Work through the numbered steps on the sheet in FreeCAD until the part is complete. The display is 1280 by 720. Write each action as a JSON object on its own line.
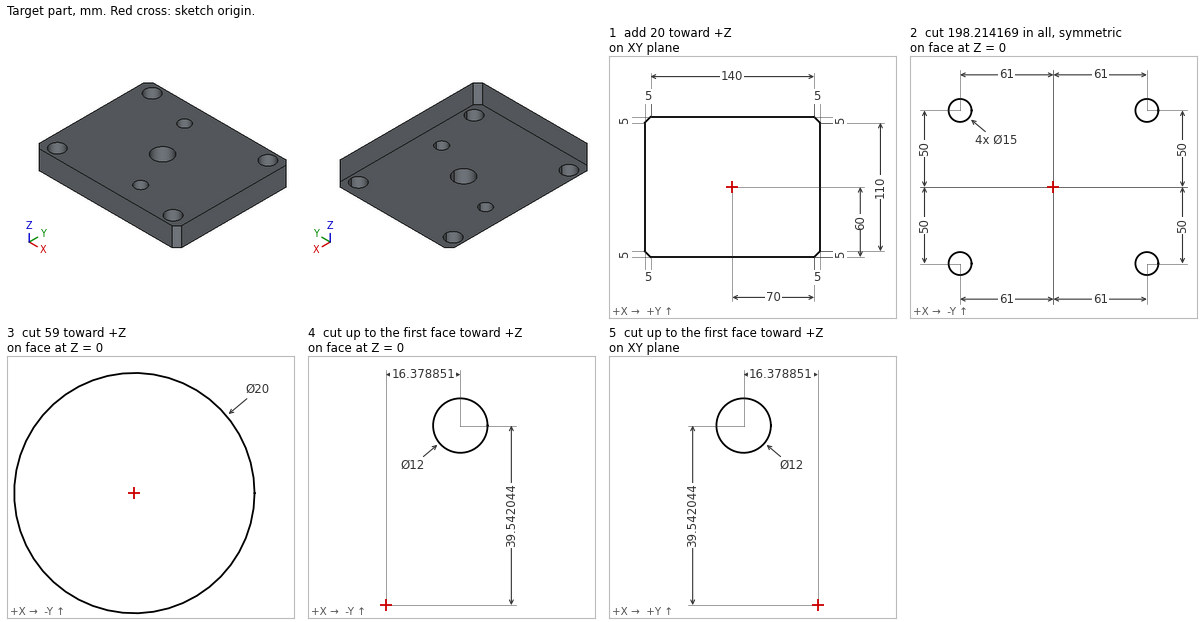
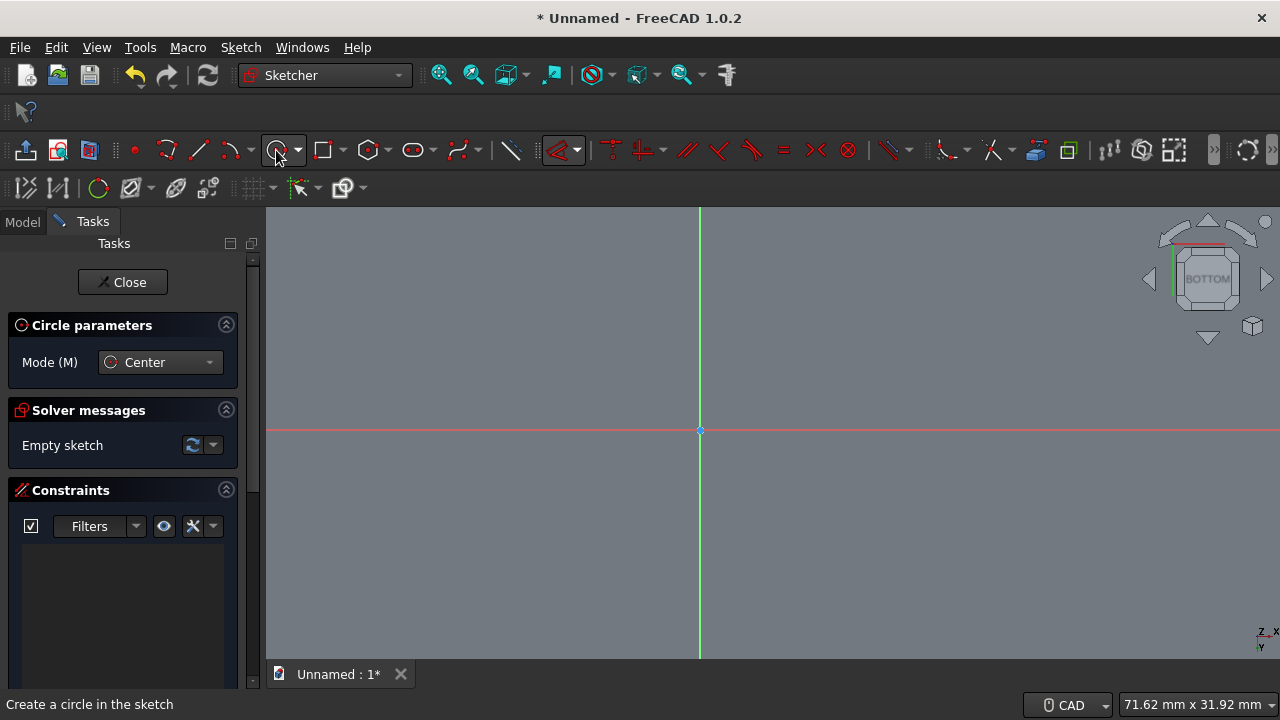
{"action": "left_click", "coordinate": [700, 430]}
{"action": "mouse_move", "coordinate": [800, 330]}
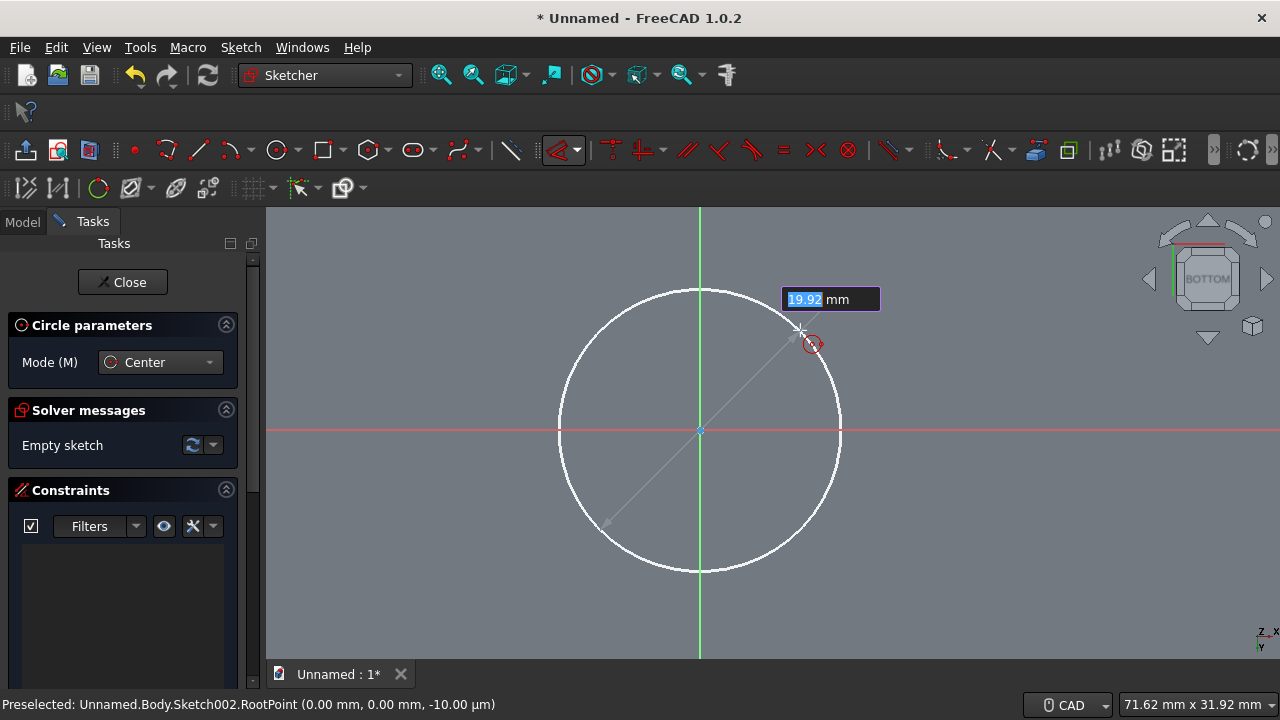
{"action": "type", "text": "20"}
{"action": "key", "text": "Return"}
{"action": "key", "text": "Escape"}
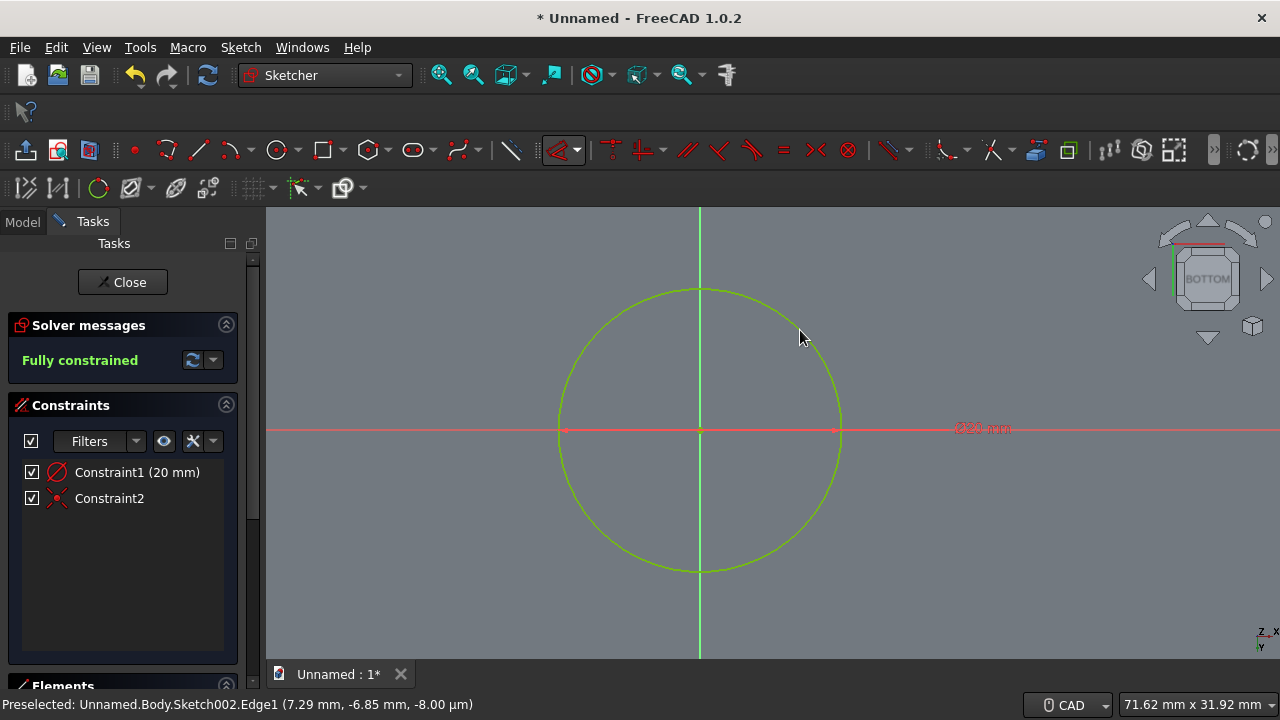
{"action": "left_click", "coordinate": [123, 282]}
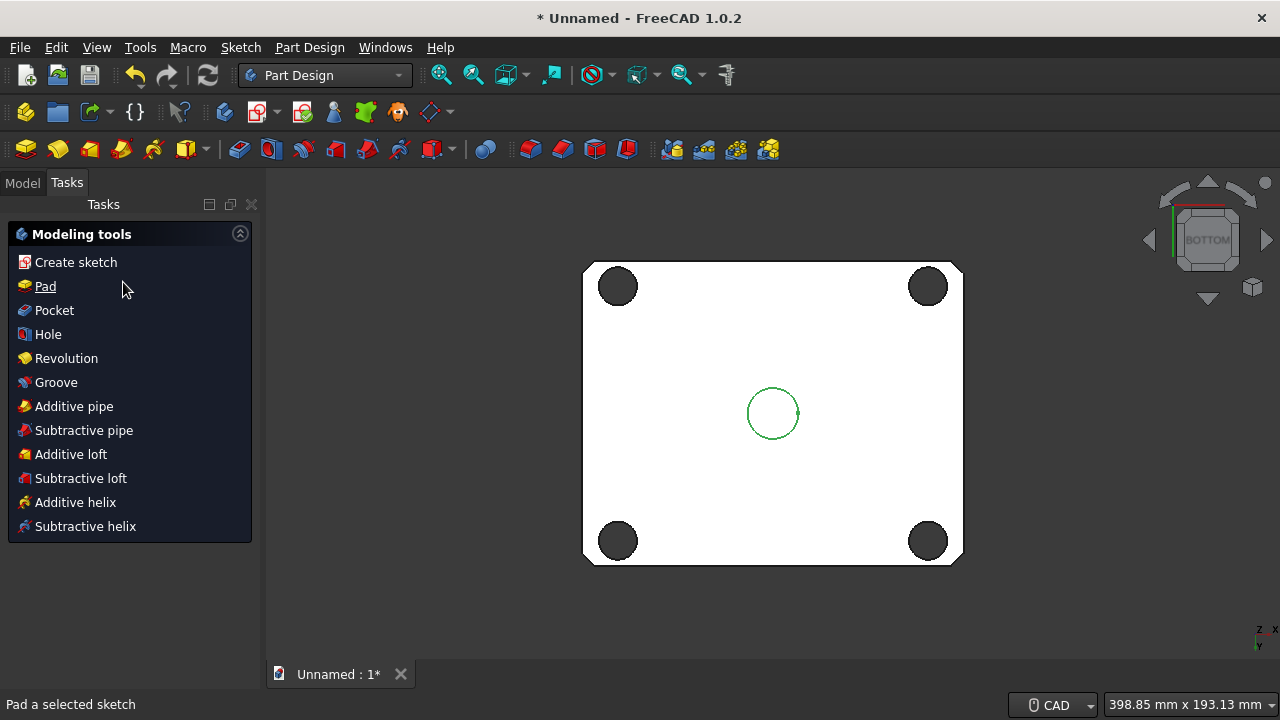
{"action": "left_click", "coordinate": [240, 150]}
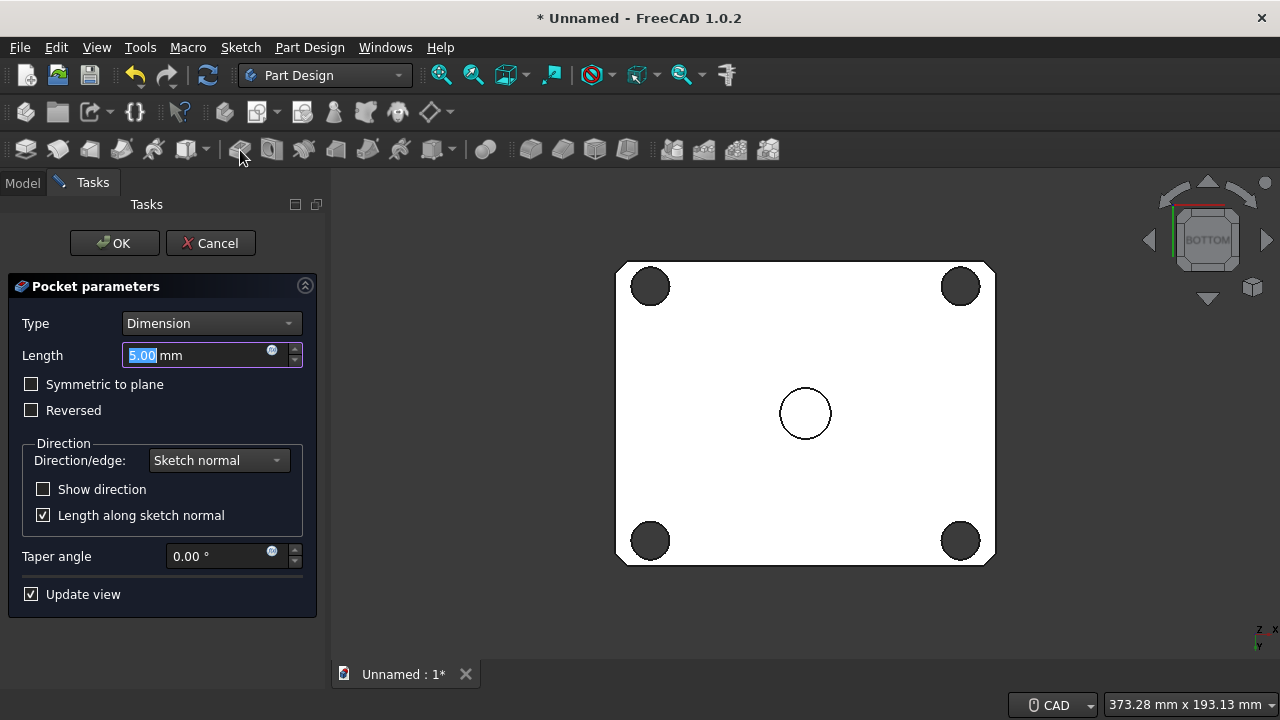
{"action": "type", "text": "59"}
{"action": "key", "text": "Tab"}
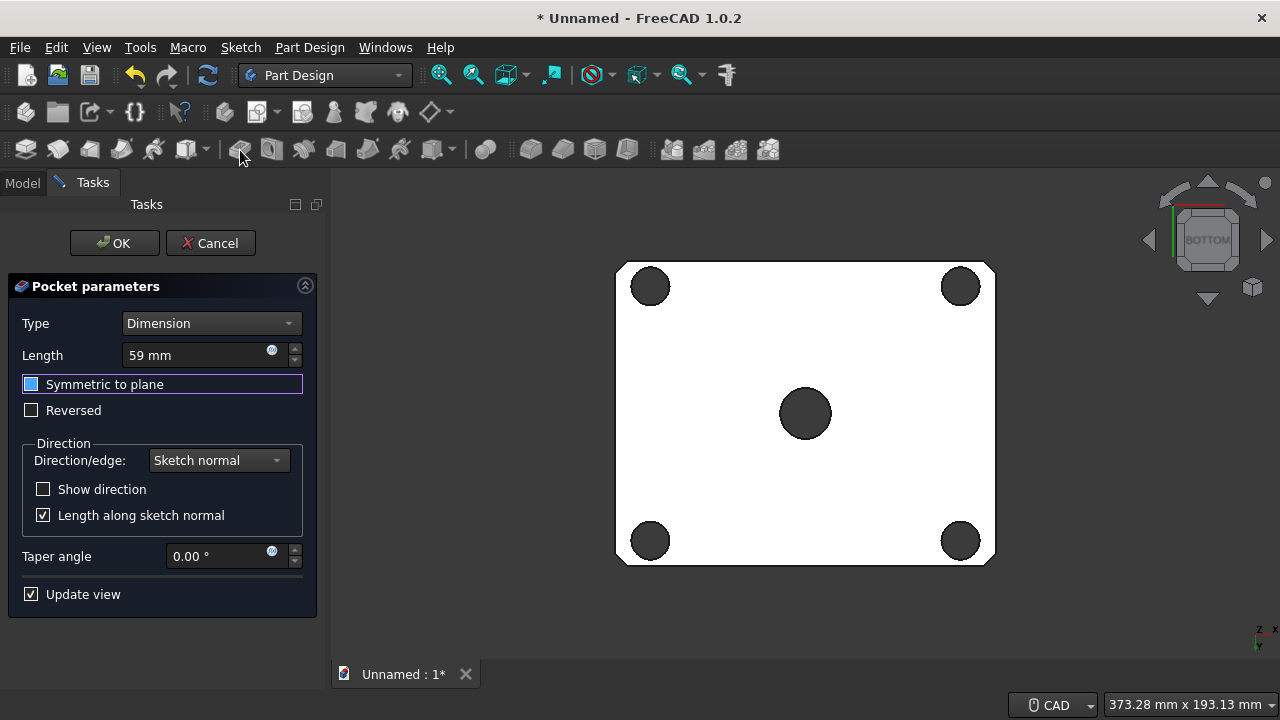
{"action": "left_click", "coordinate": [115, 243]}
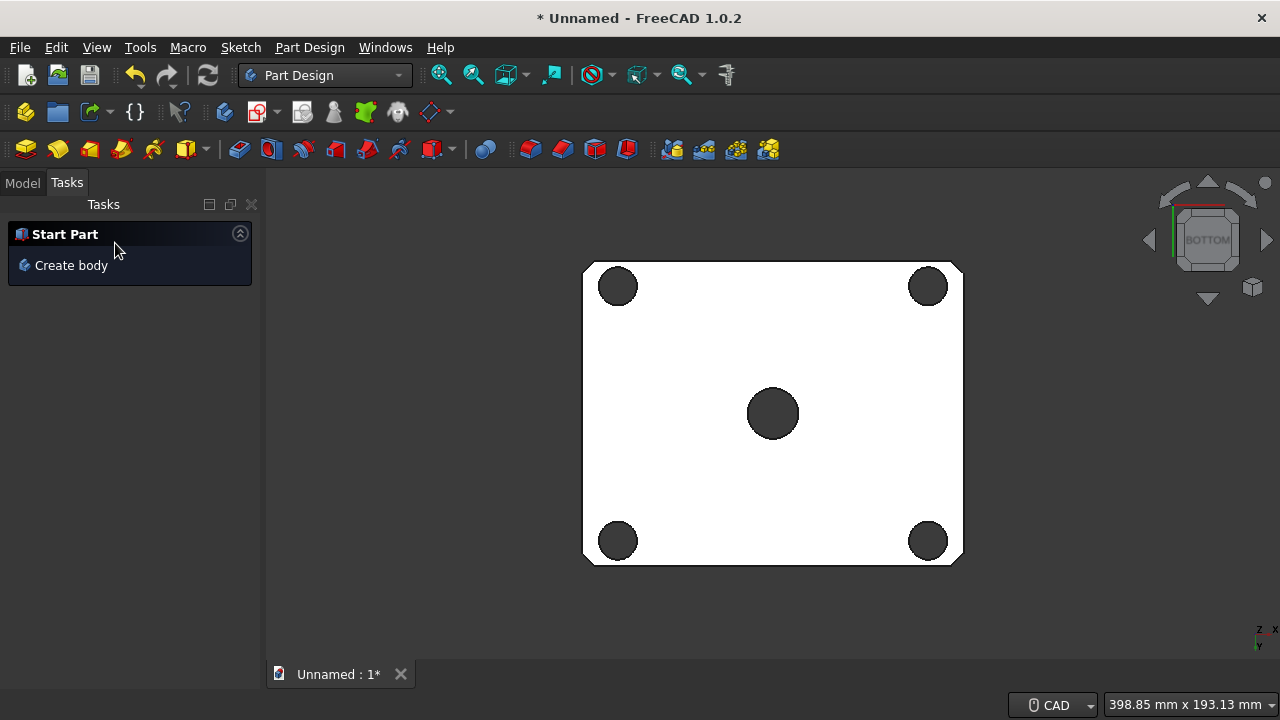
{"action": "left_click", "coordinate": [664, 413]}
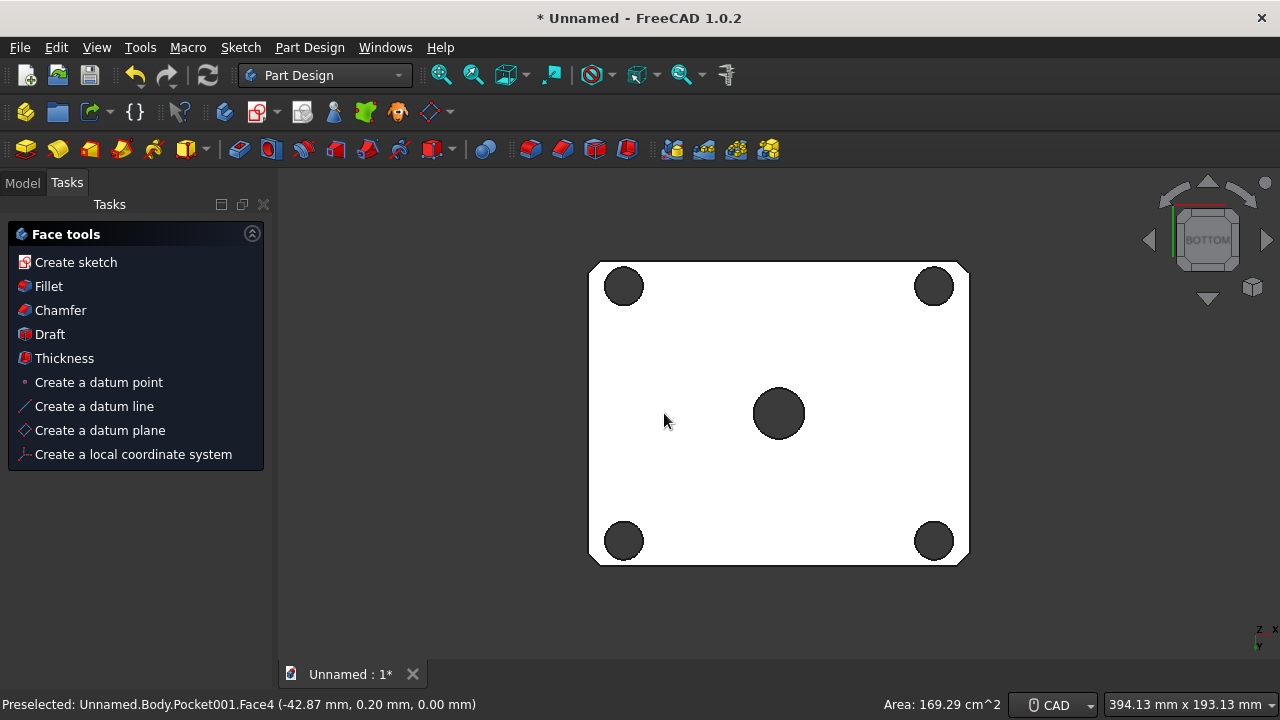
{"action": "left_click", "coordinate": [258, 112]}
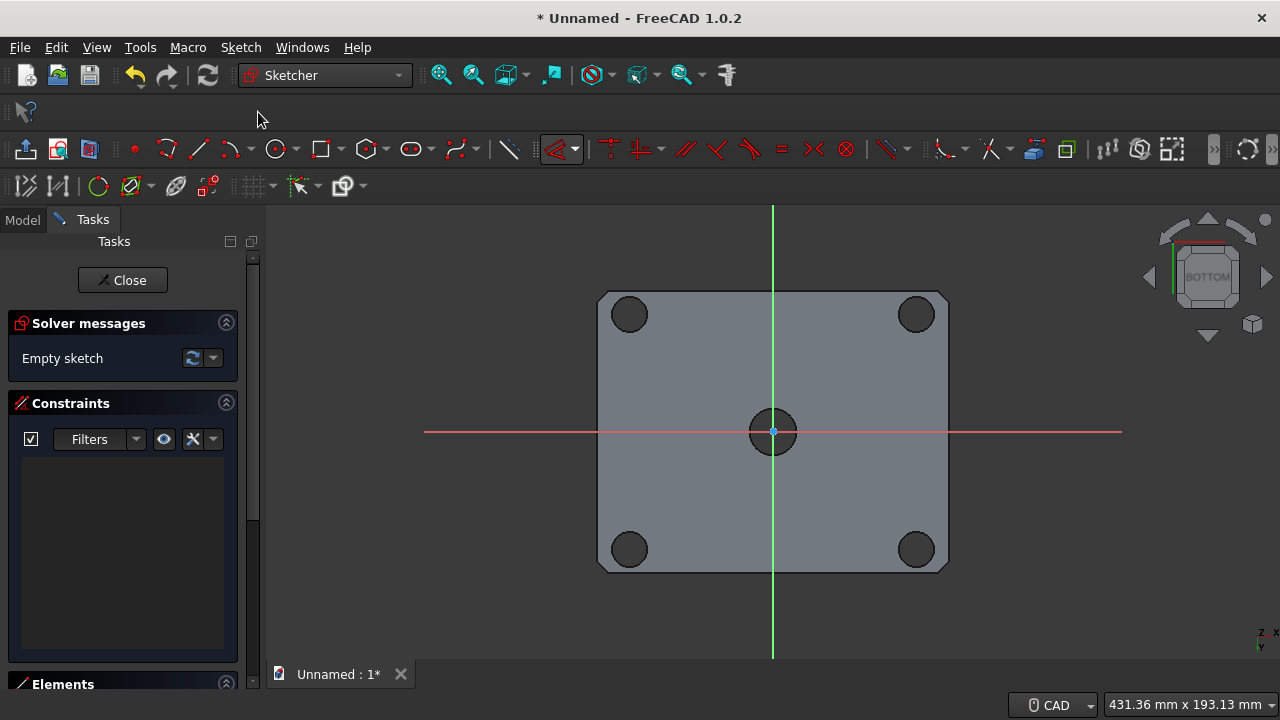
{"action": "scroll", "coordinate": [825, 327], "scroll_direction": "up", "scroll_amount": 11}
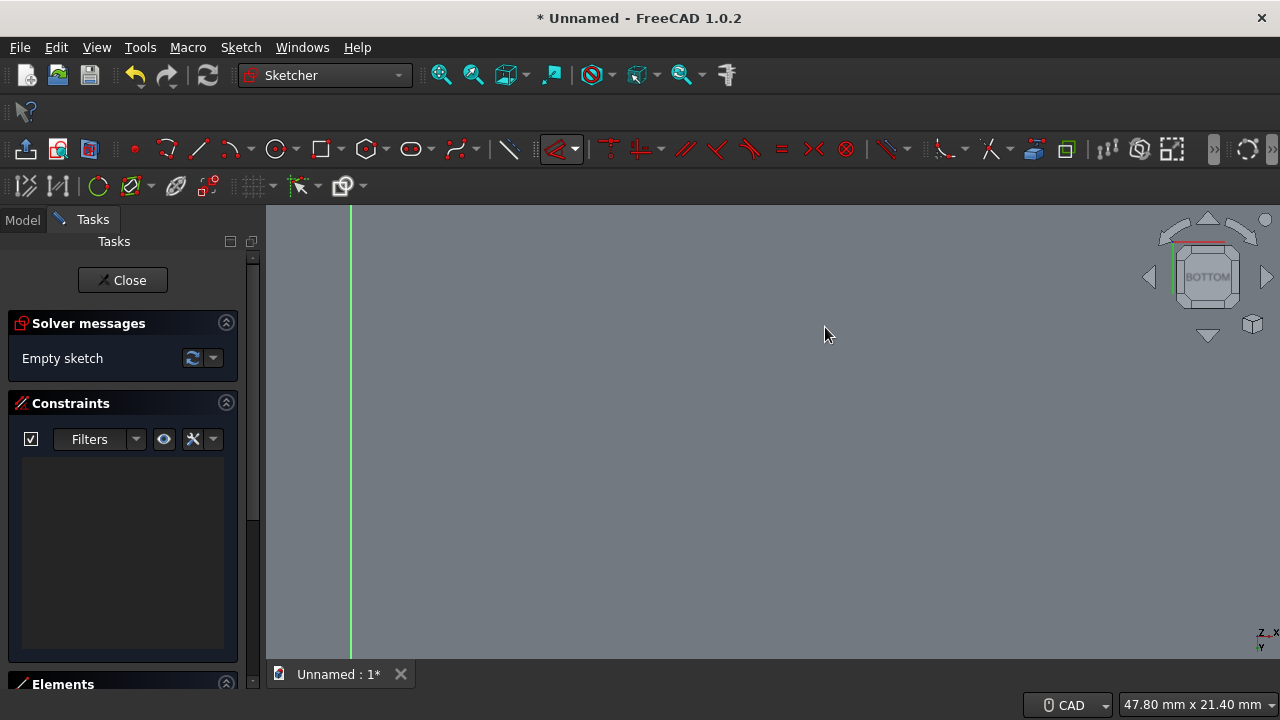
{"action": "left_click", "coordinate": [276, 150]}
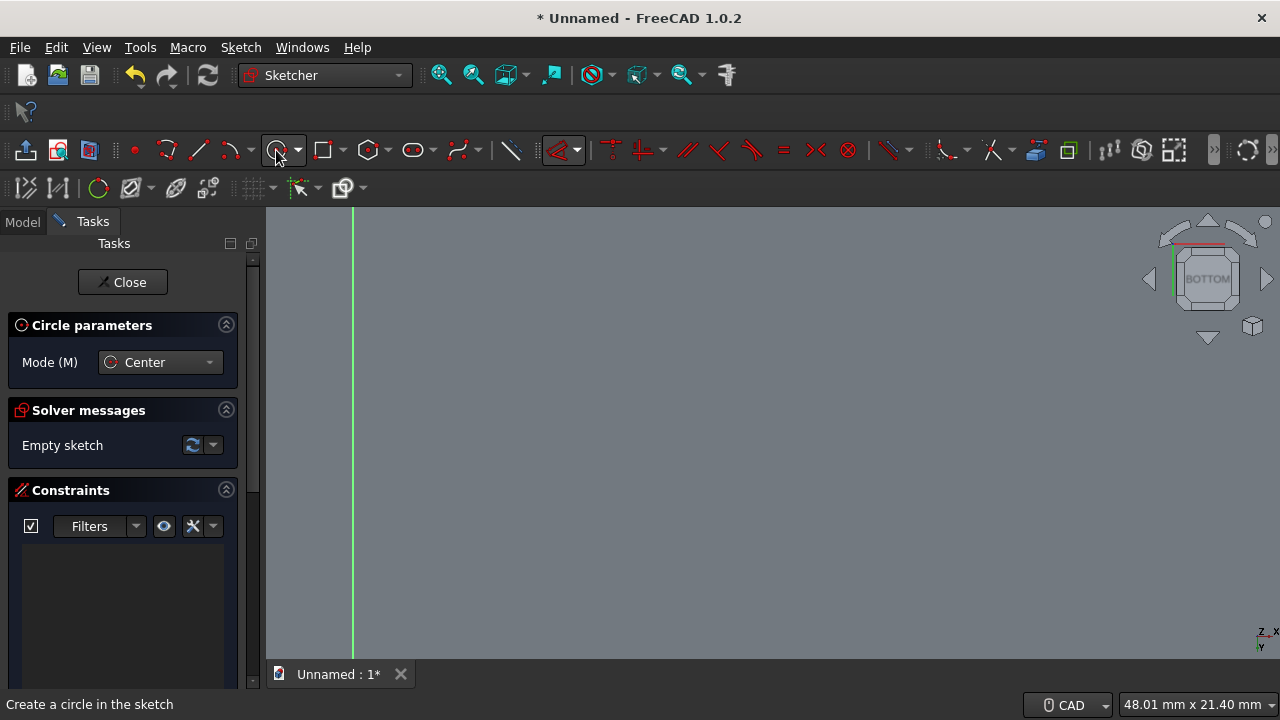
{"action": "left_click", "coordinate": [699, 435]}
{"action": "mouse_move", "coordinate": [789, 345]}